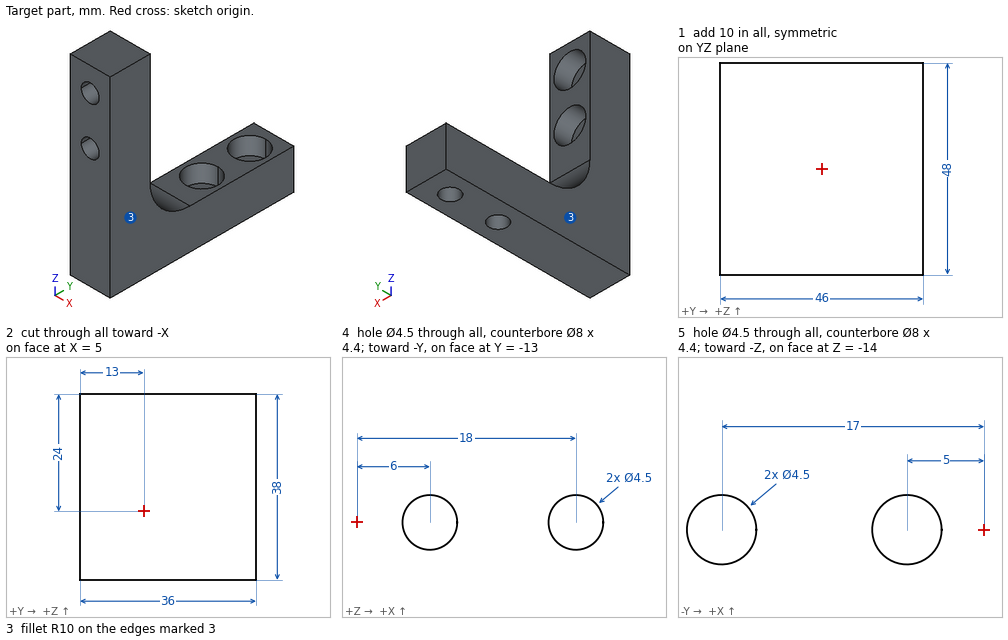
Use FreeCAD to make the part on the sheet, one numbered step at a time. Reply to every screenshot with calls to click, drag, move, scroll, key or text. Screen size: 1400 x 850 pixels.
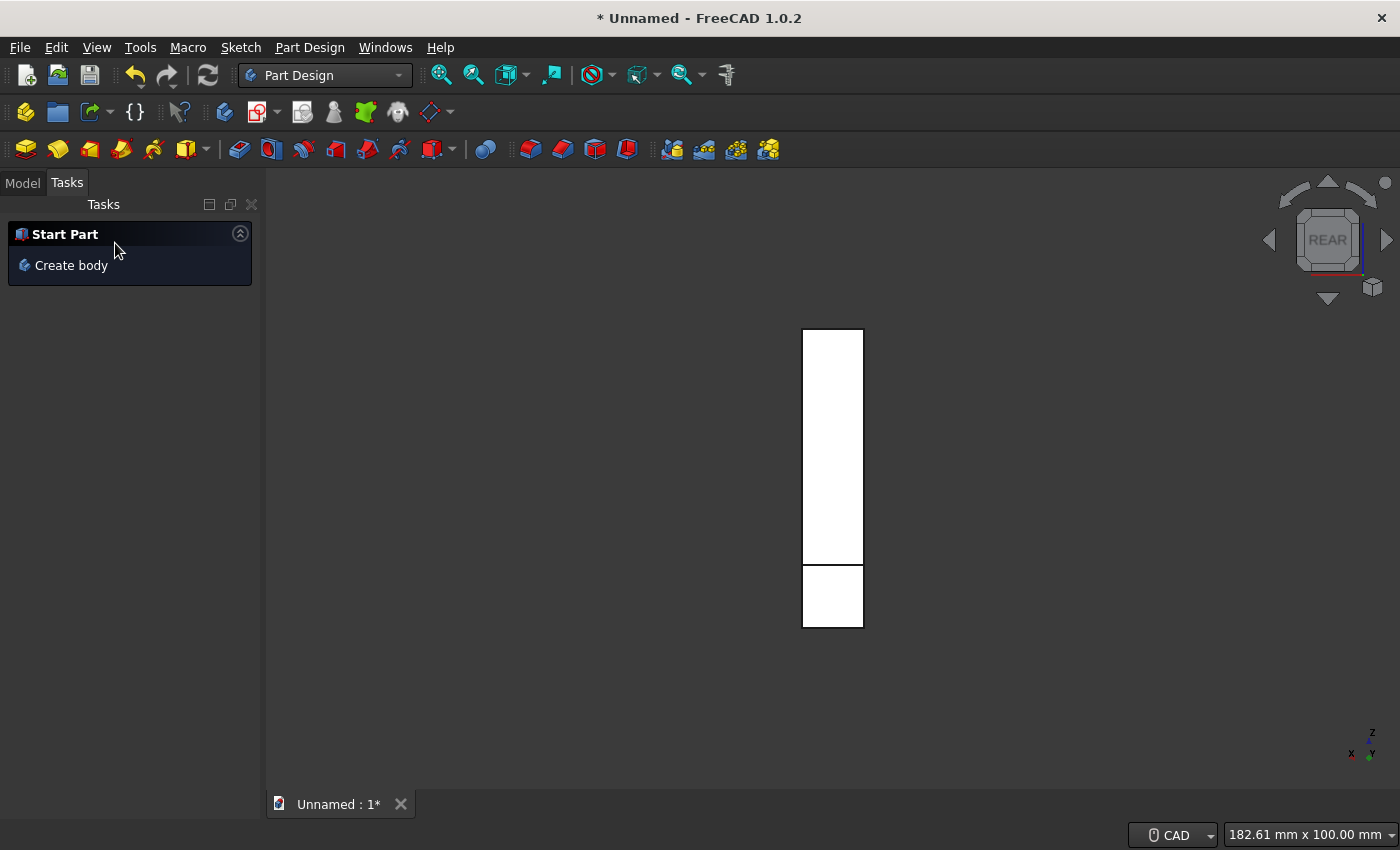
key(6)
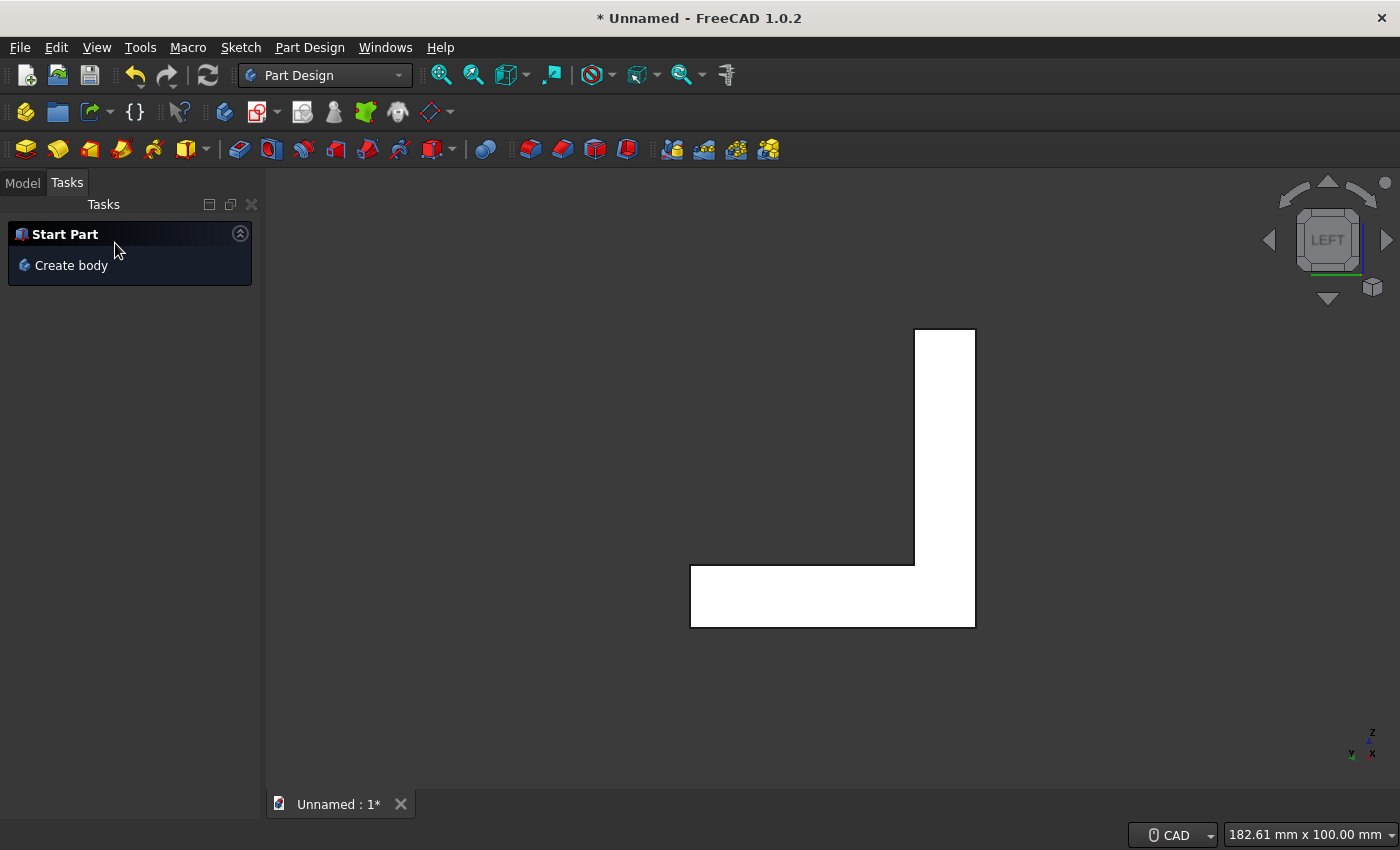
key(v)
key(3)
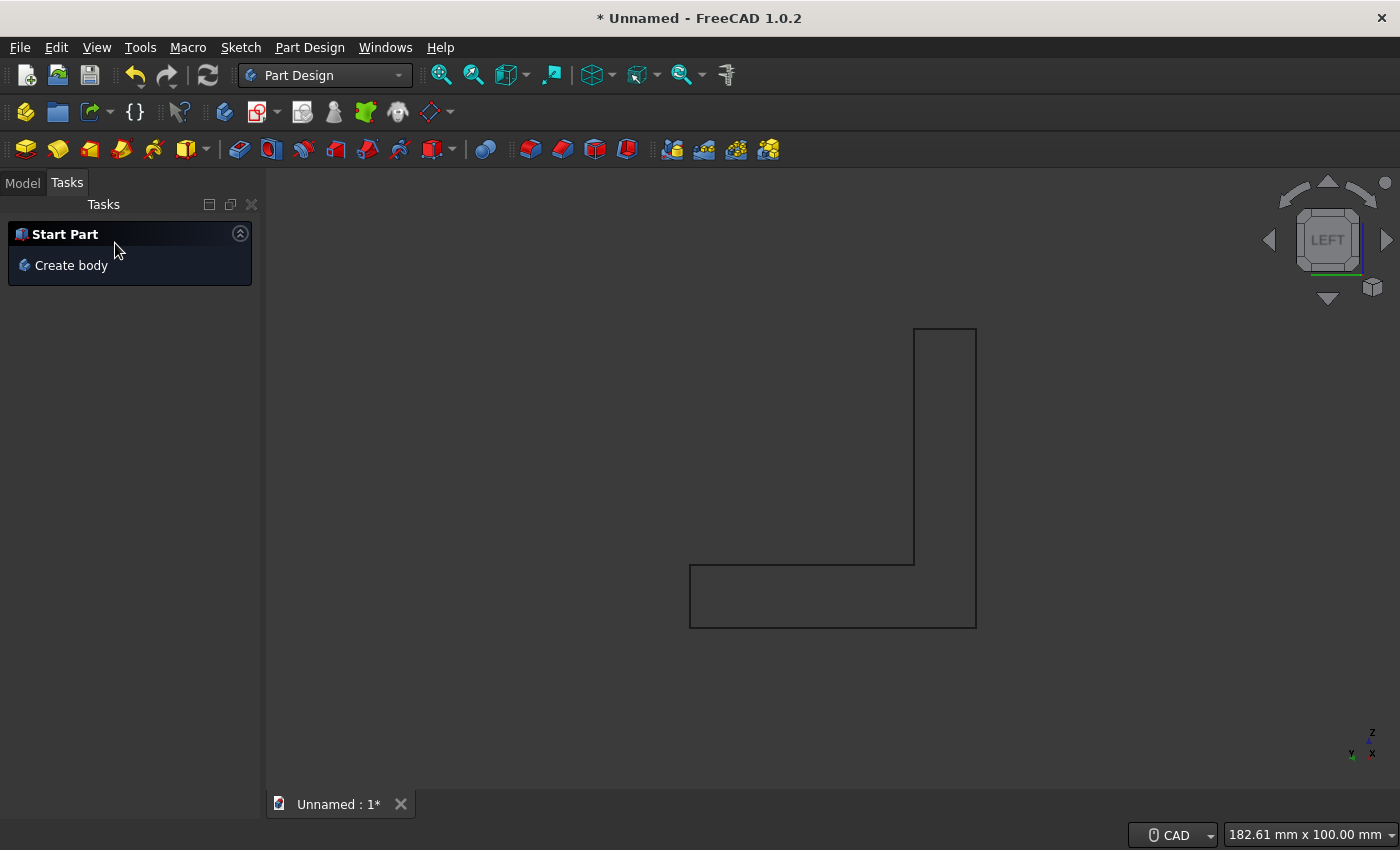
key(0)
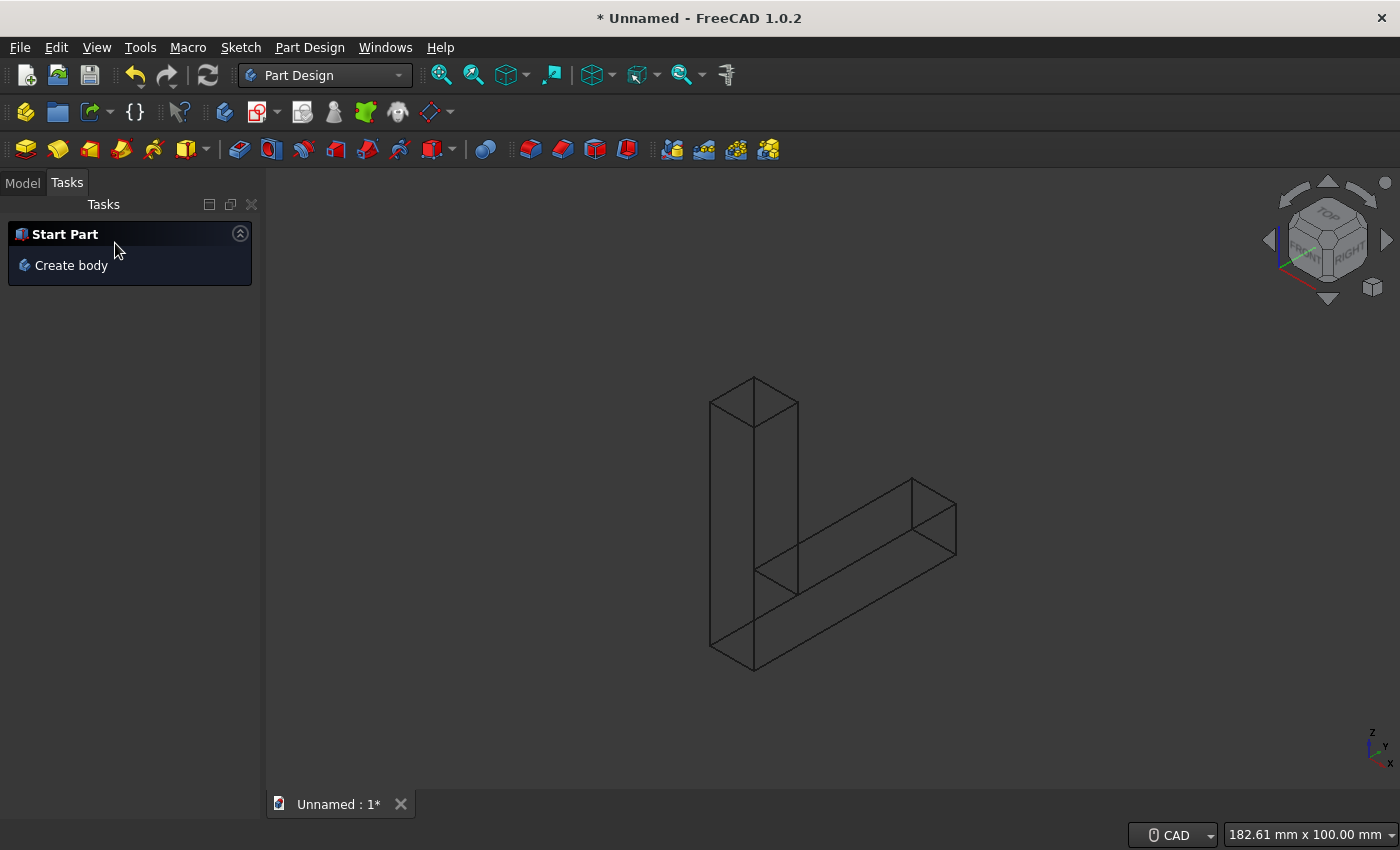
click(776, 581)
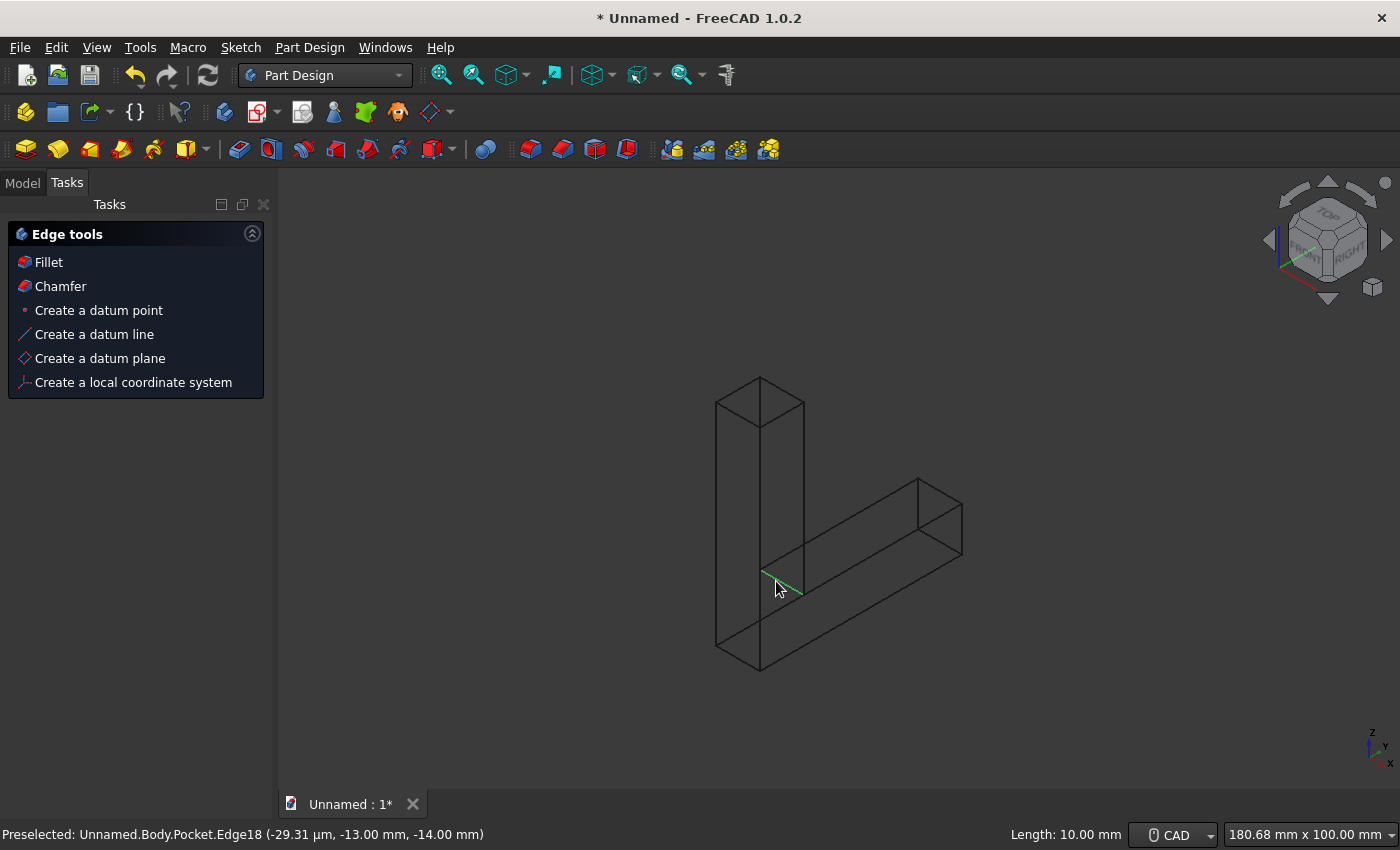
key(v)
key(1)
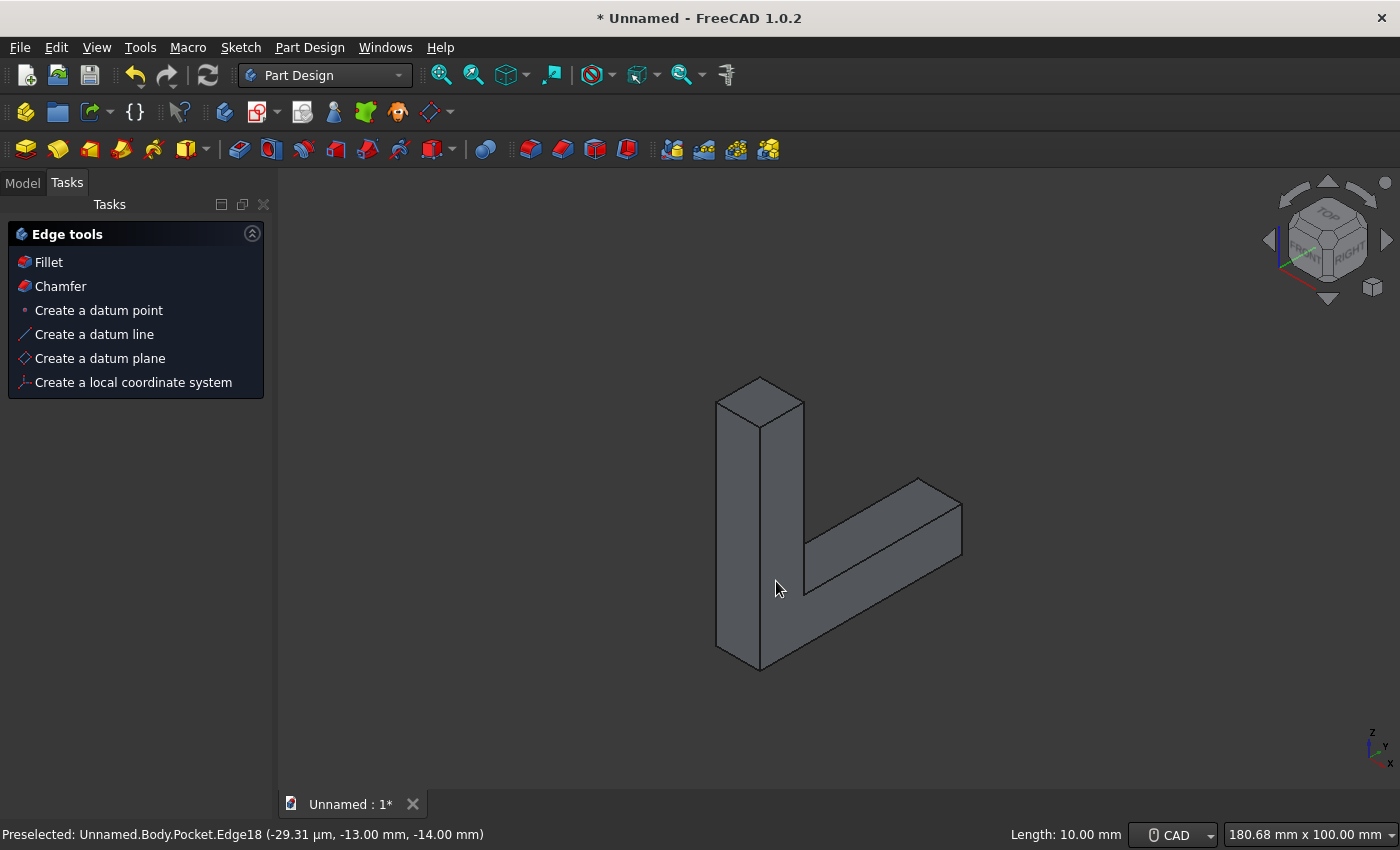
click(532, 150)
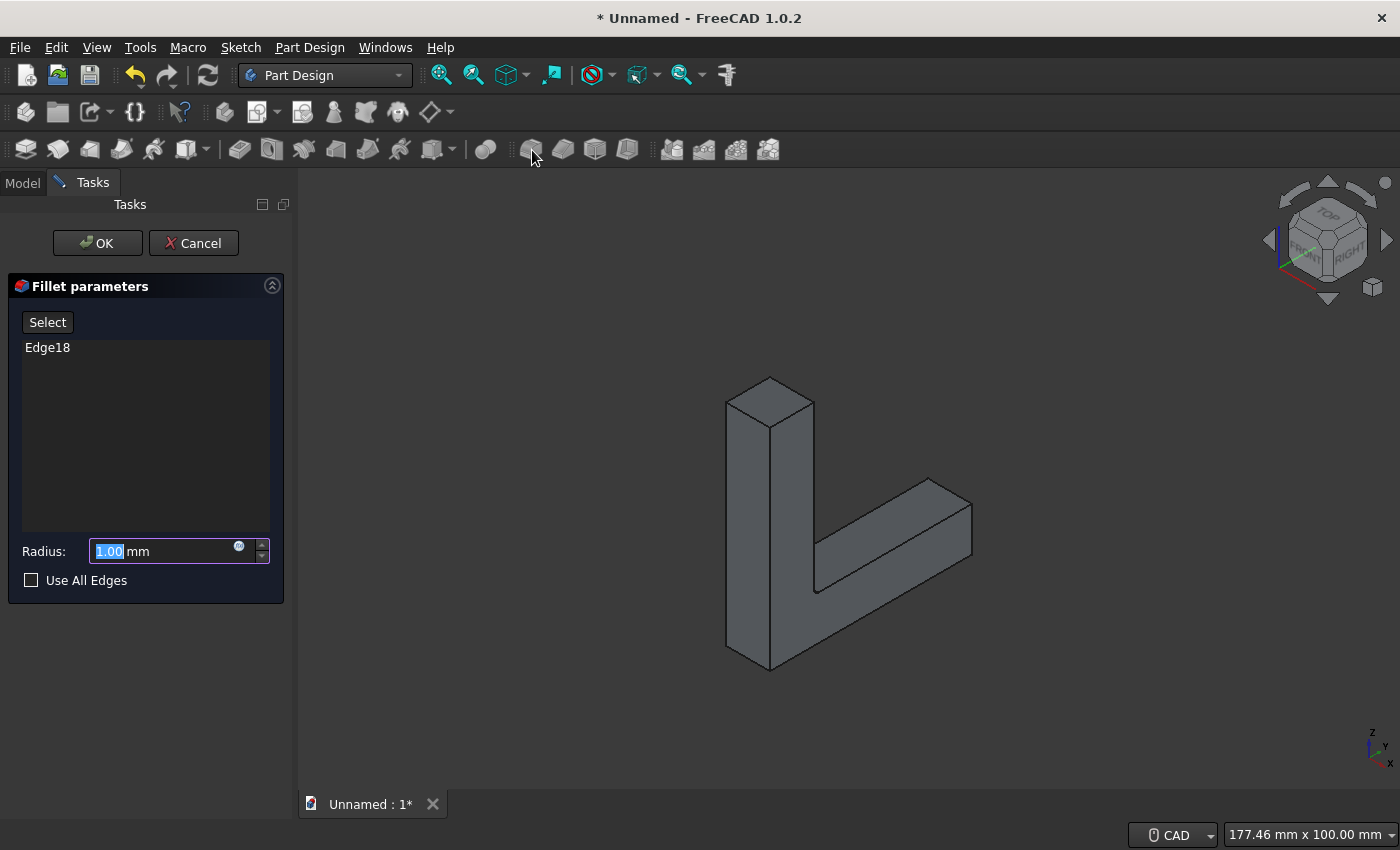
text(10)
key(Tab)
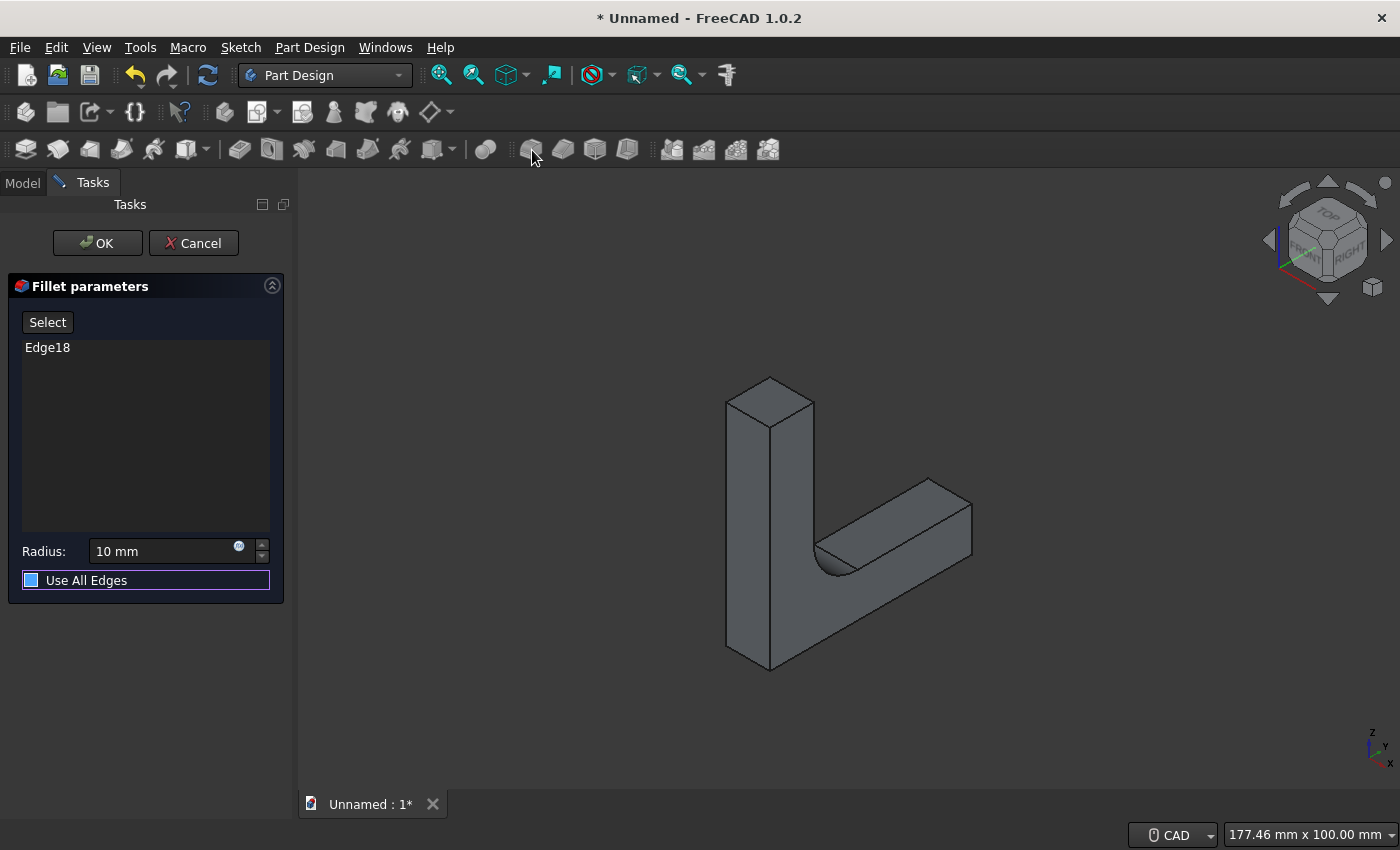
click(98, 243)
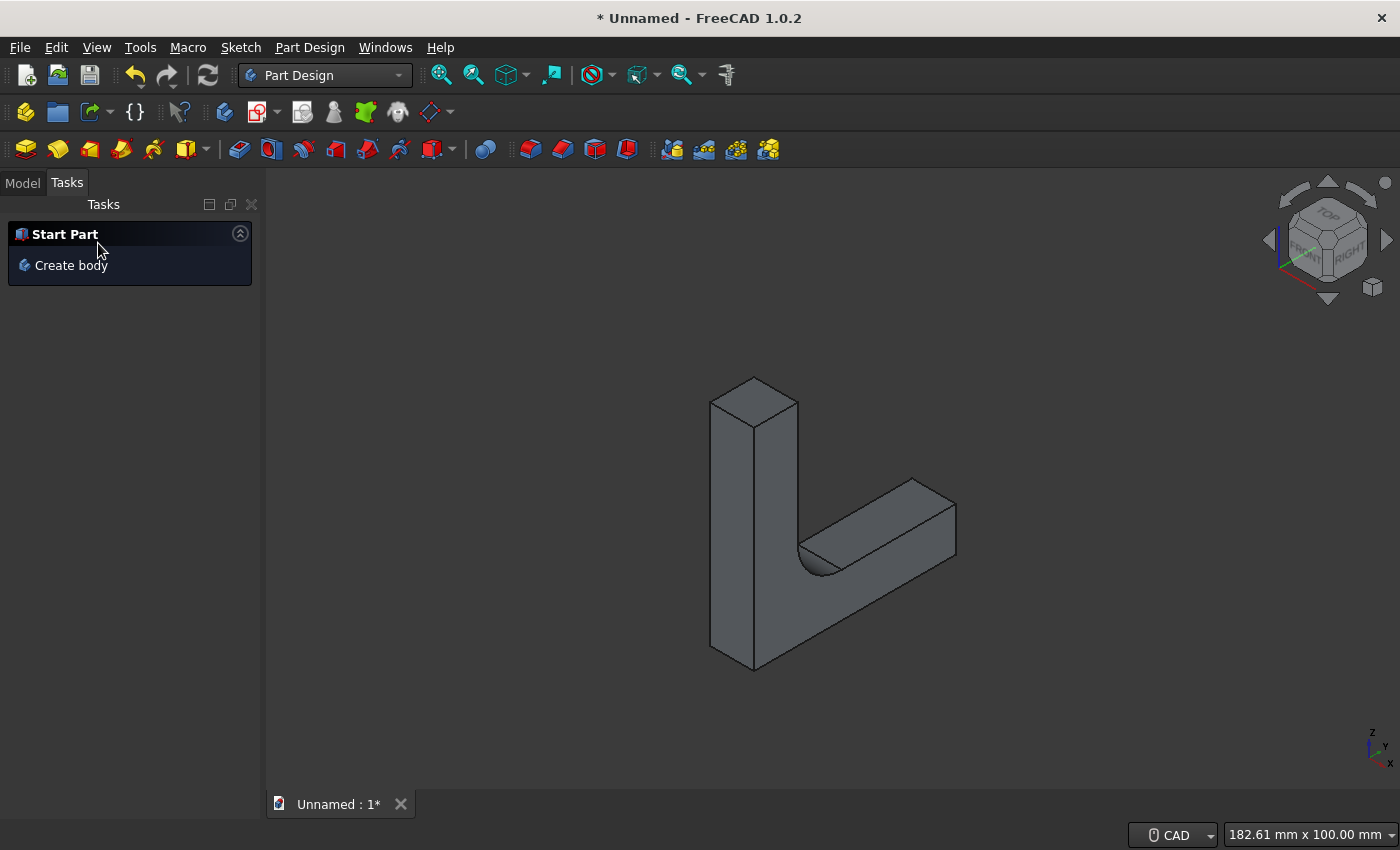
key(4)